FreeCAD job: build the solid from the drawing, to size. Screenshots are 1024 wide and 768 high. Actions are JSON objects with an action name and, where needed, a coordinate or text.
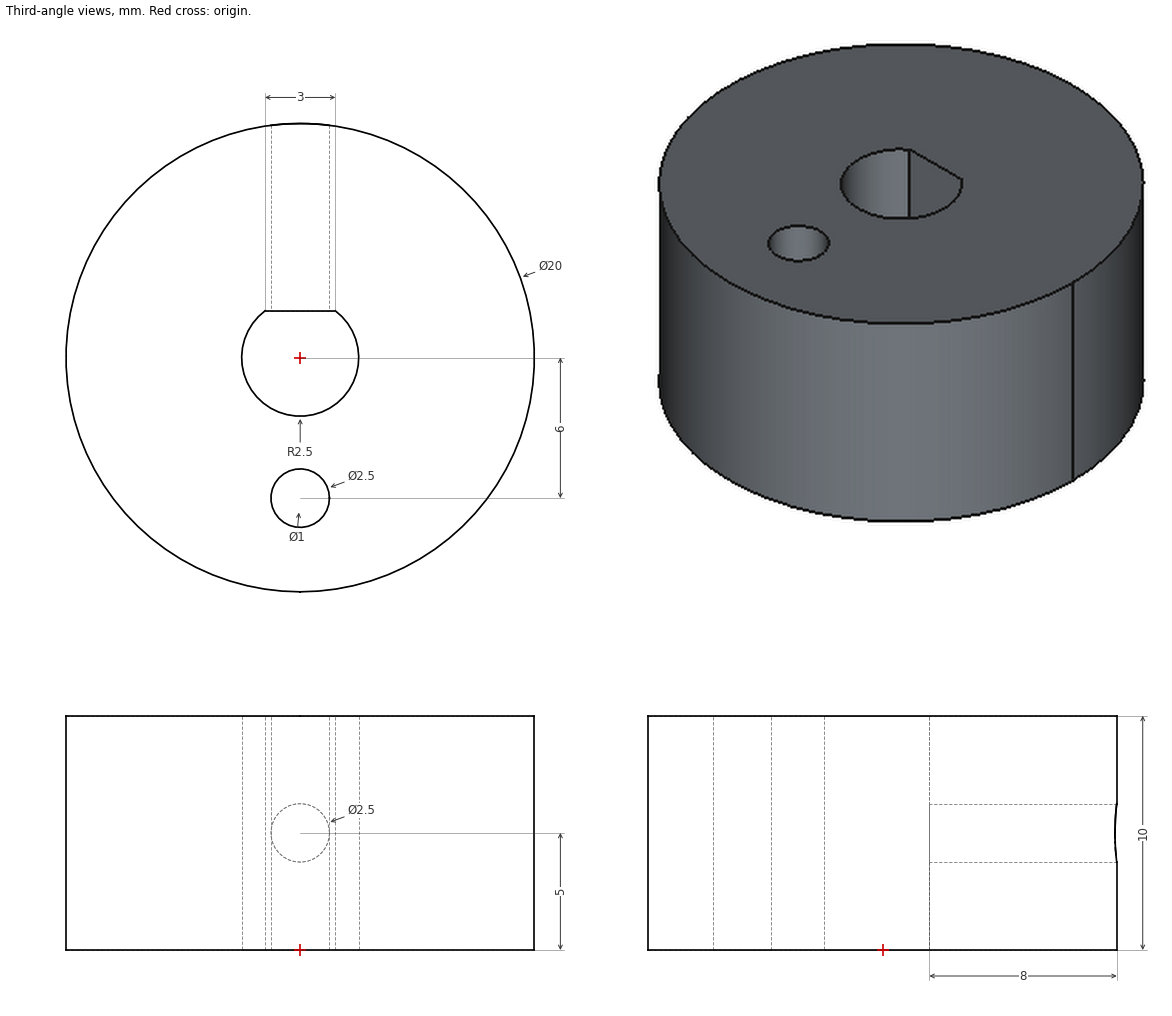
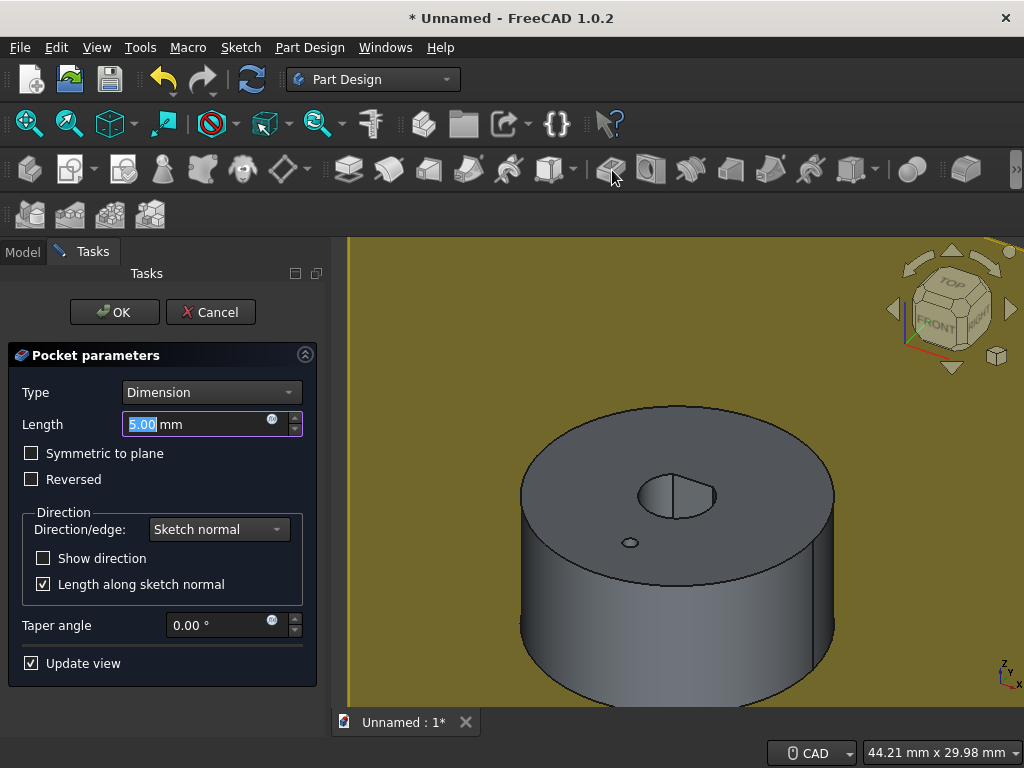
{"action": "type", "text": "8"}
{"action": "key", "text": "Tab"}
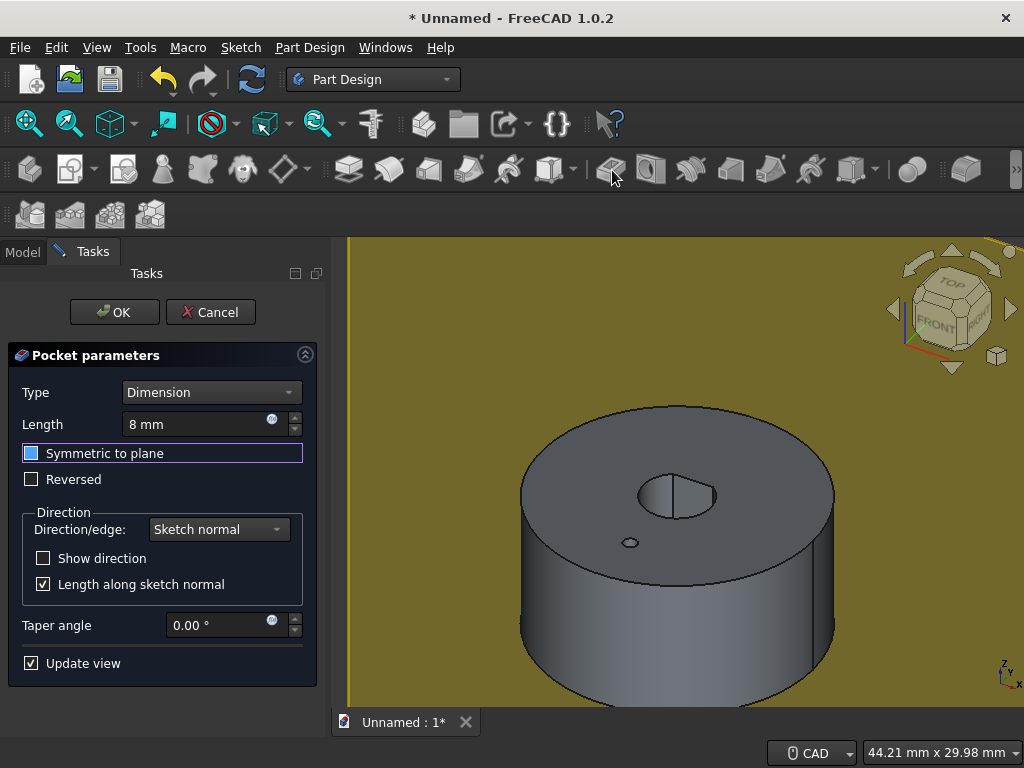
{"action": "left_click", "coordinate": [30, 479]}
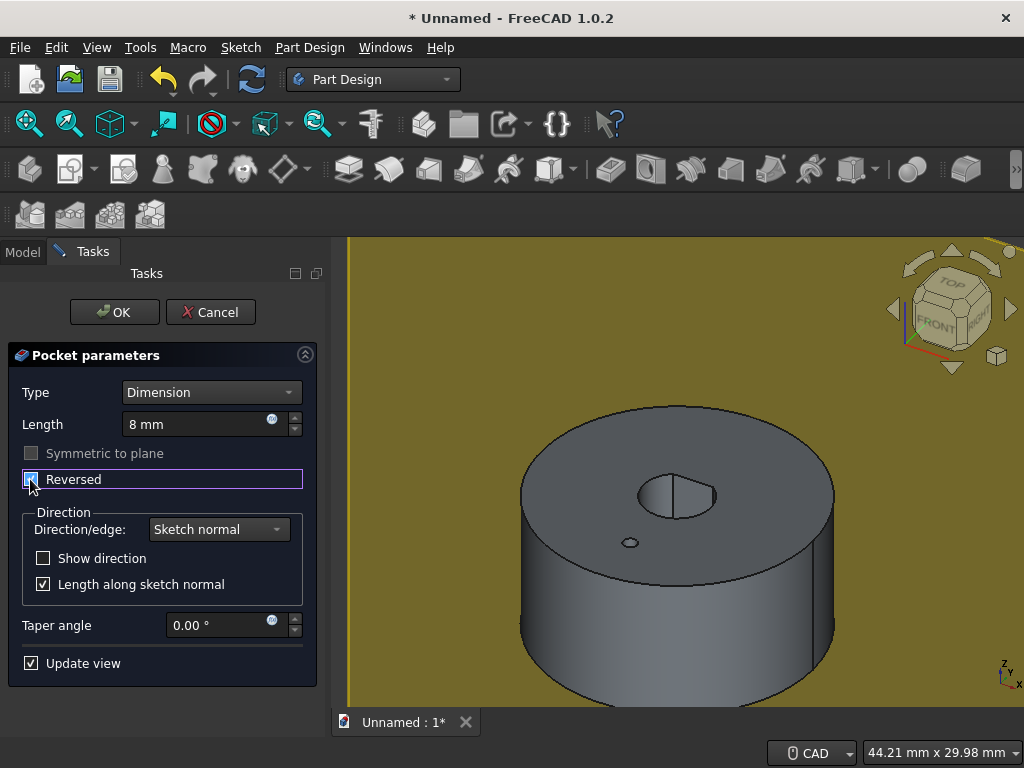
{"action": "left_click", "coordinate": [115, 312]}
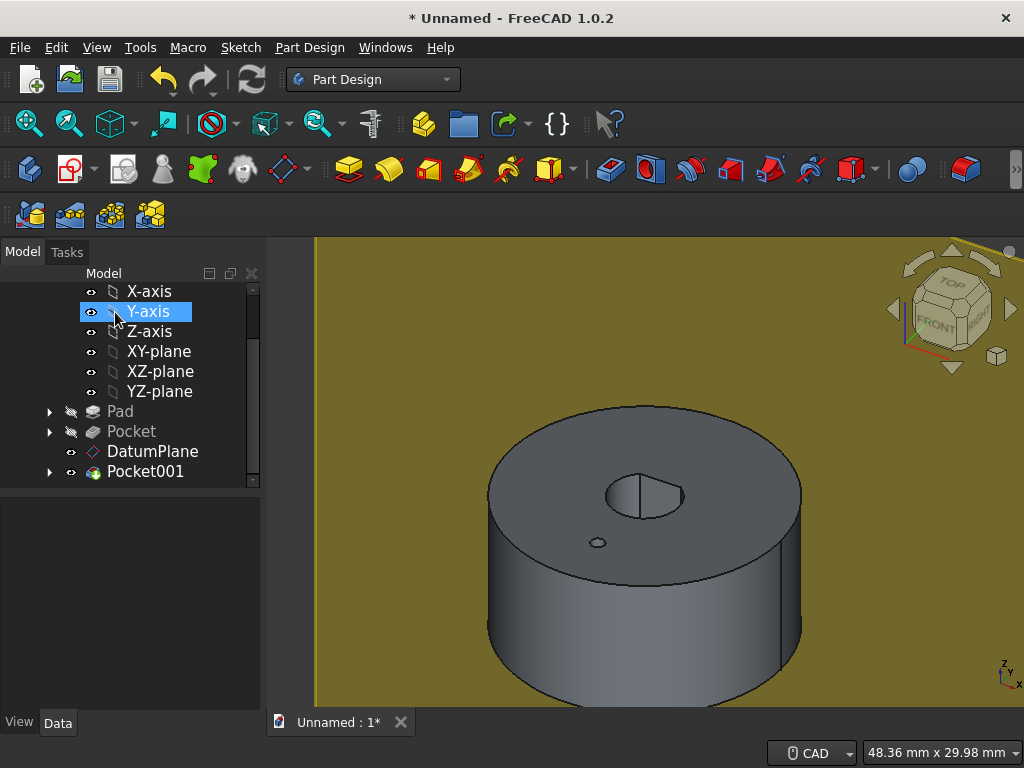
{"action": "left_click", "coordinate": [116, 452]}
{"action": "key", "text": "space"}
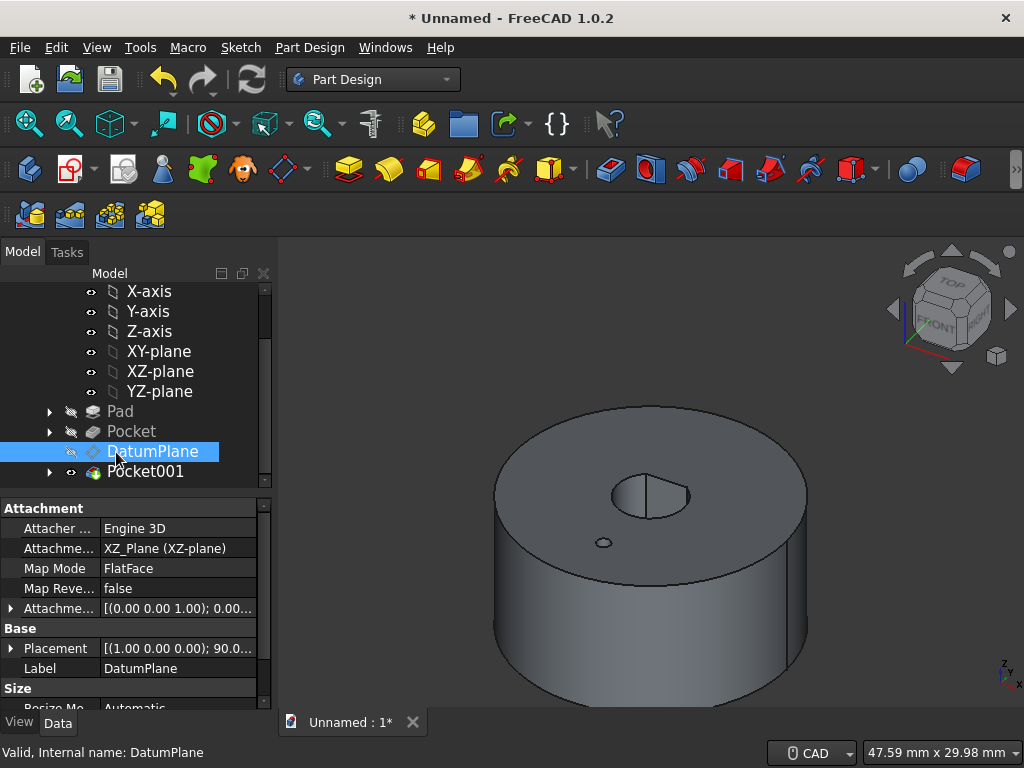
{"action": "key", "text": "v f"}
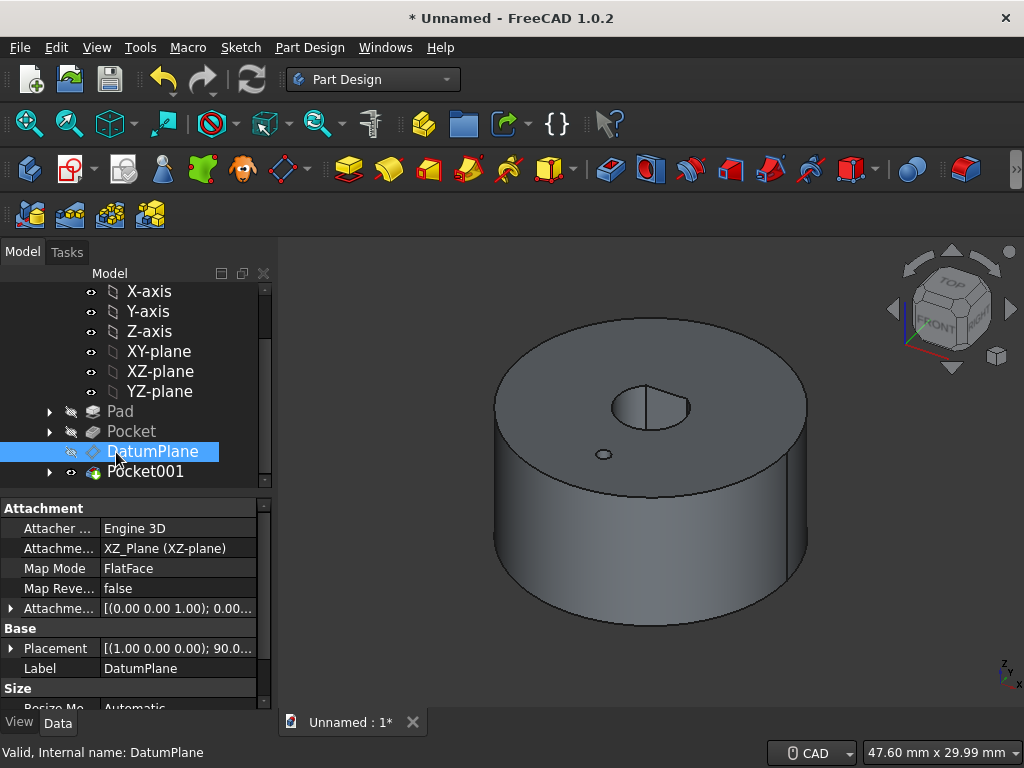
{"action": "key", "text": "5"}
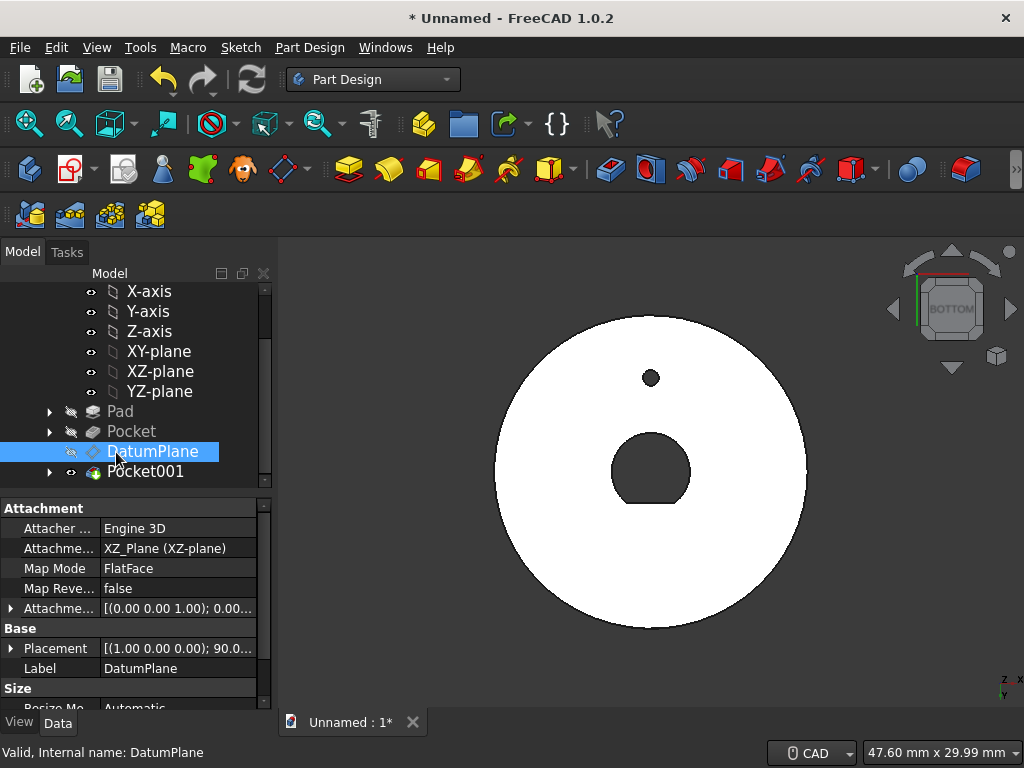
{"action": "left_click", "coordinate": [651, 561]}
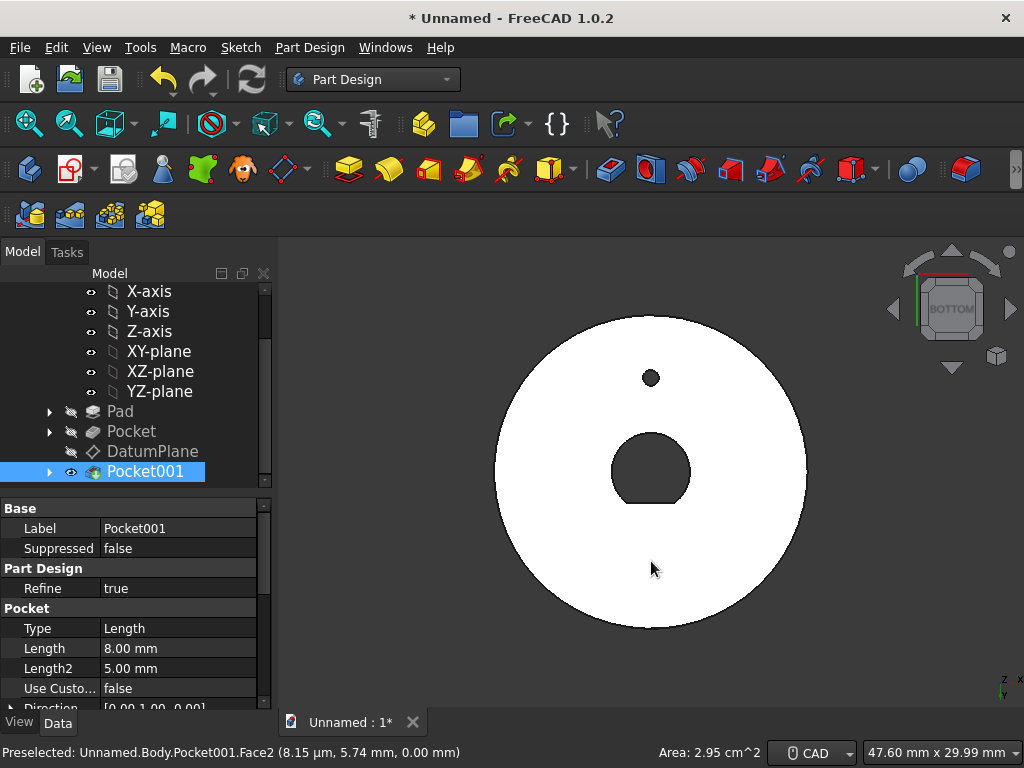
{"action": "left_click", "coordinate": [70, 170]}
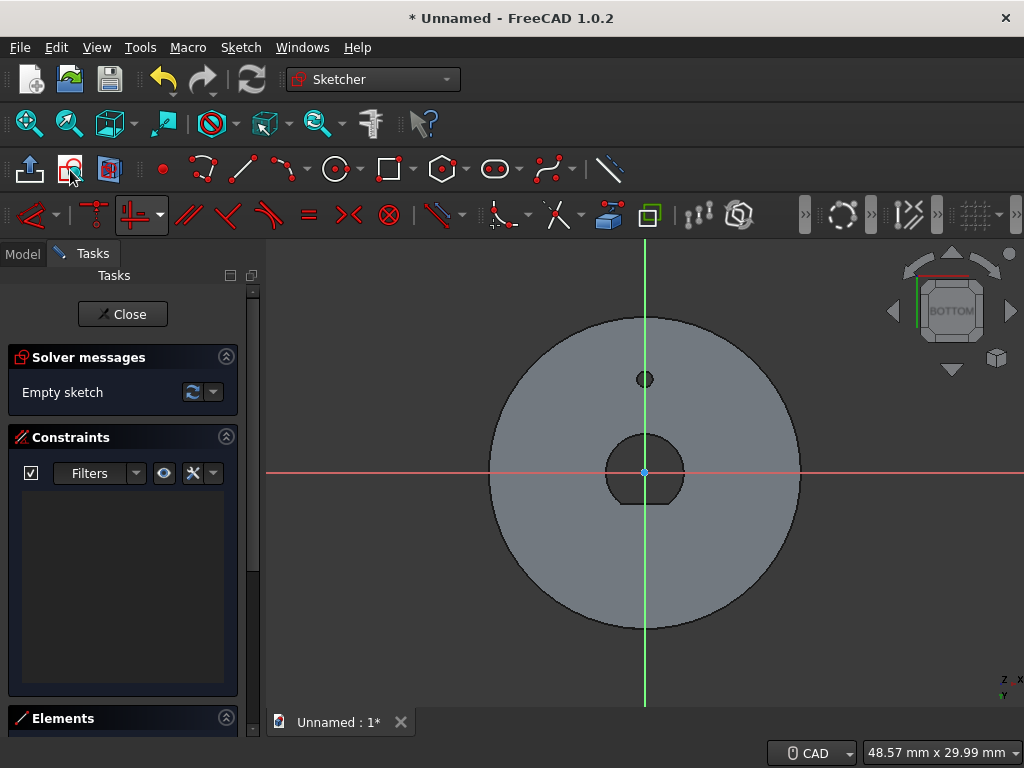
{"action": "scroll", "coordinate": [656, 365], "scroll_direction": "up", "scroll_amount": 10}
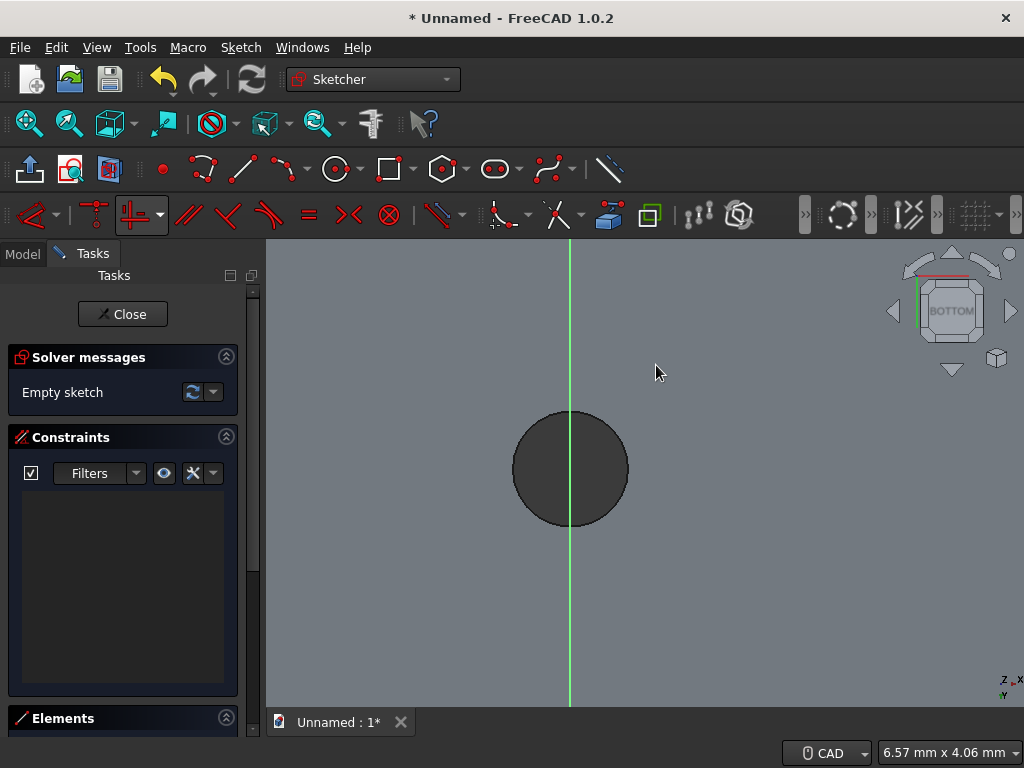
{"action": "key", "text": "g c"}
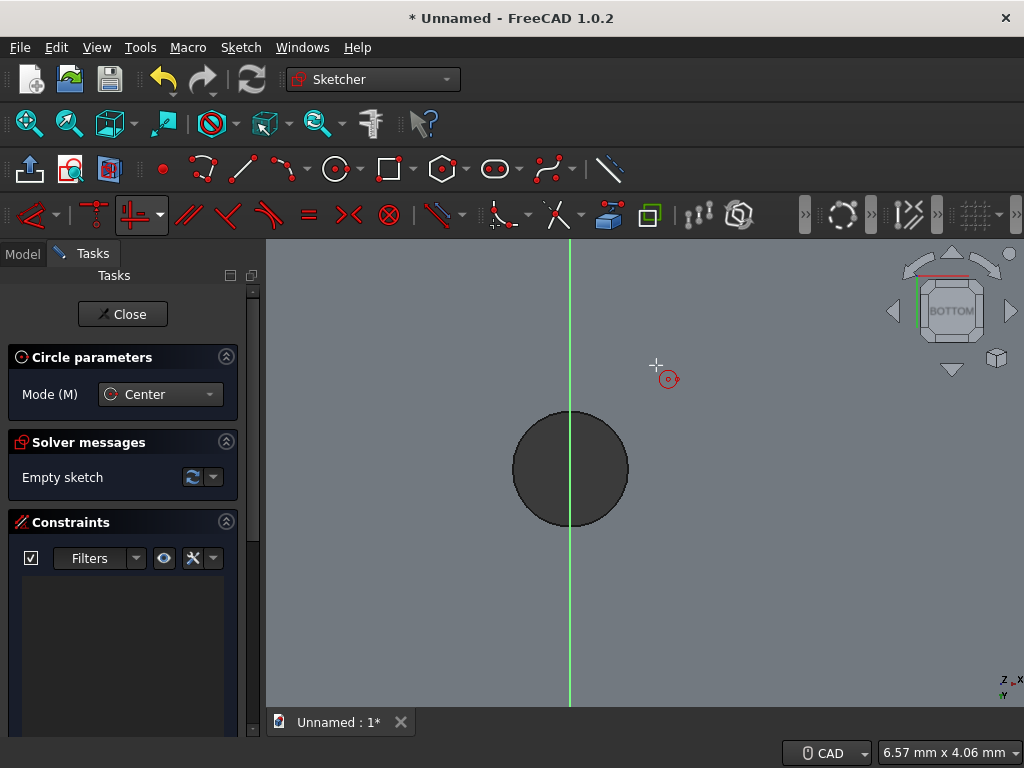
{"action": "left_click", "coordinate": [570, 469]}
{"action": "mouse_move", "coordinate": [672, 367]}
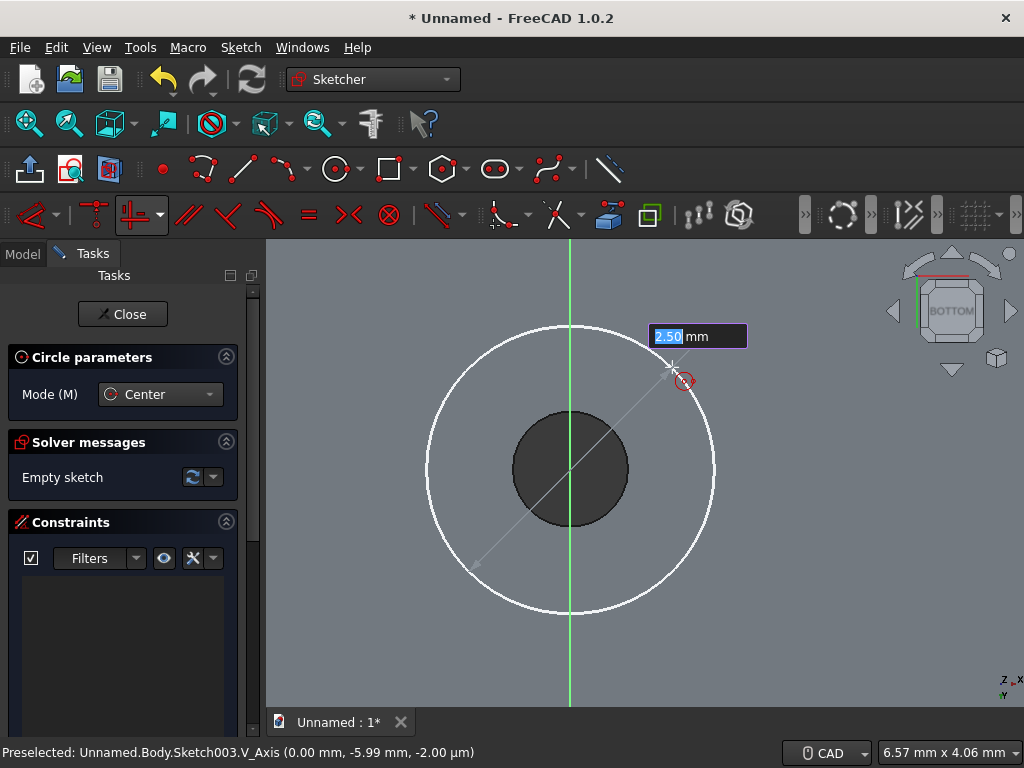
{"action": "type", "text": "2.5"}
{"action": "key", "text": "Return"}
{"action": "key", "text": "Escape"}